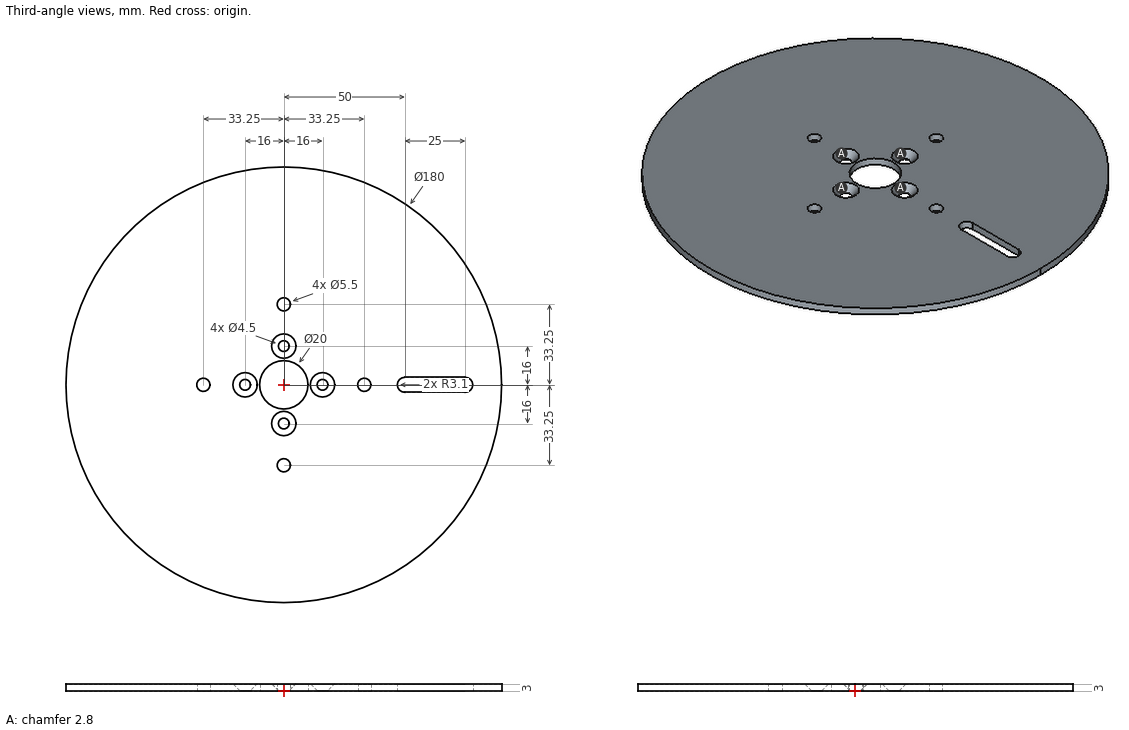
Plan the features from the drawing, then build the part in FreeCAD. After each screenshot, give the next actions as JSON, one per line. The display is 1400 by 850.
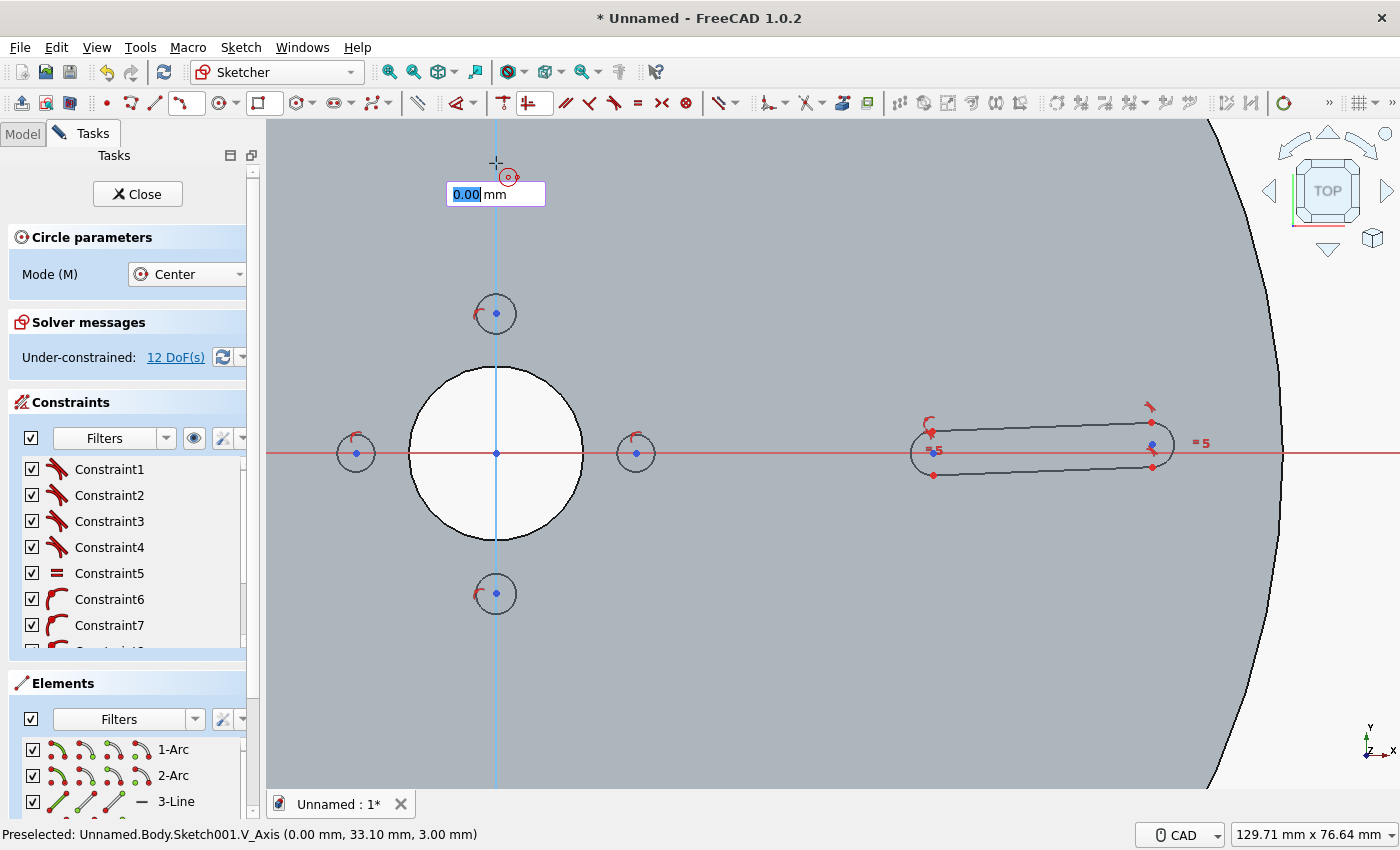
{"action": "scroll", "coordinate": [936, 455], "scroll_direction": "down", "scroll_amount": 2}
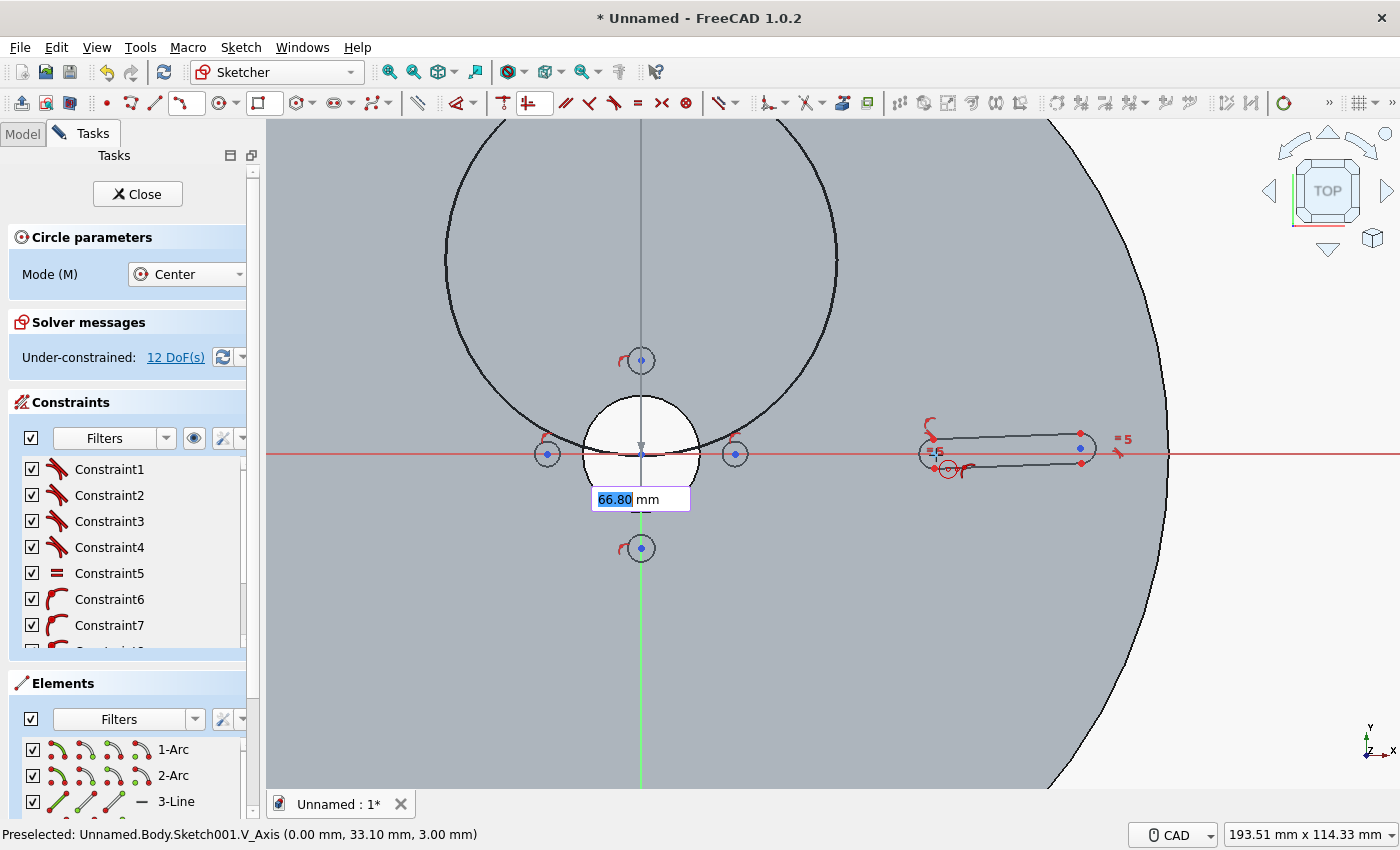
{"action": "scroll", "coordinate": [653, 248], "scroll_direction": "up", "scroll_amount": 2}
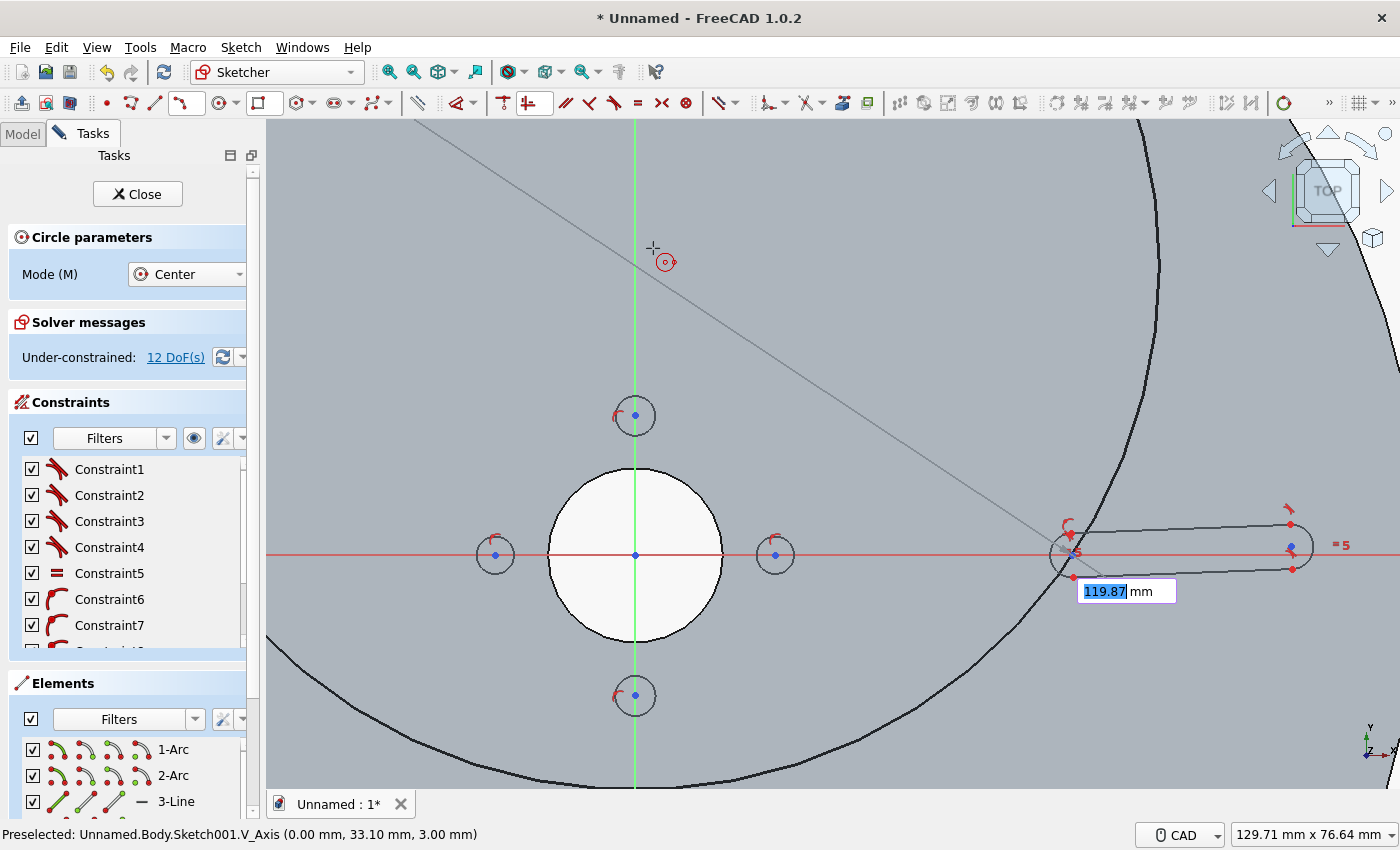
{"action": "left_click", "coordinate": [652, 248]}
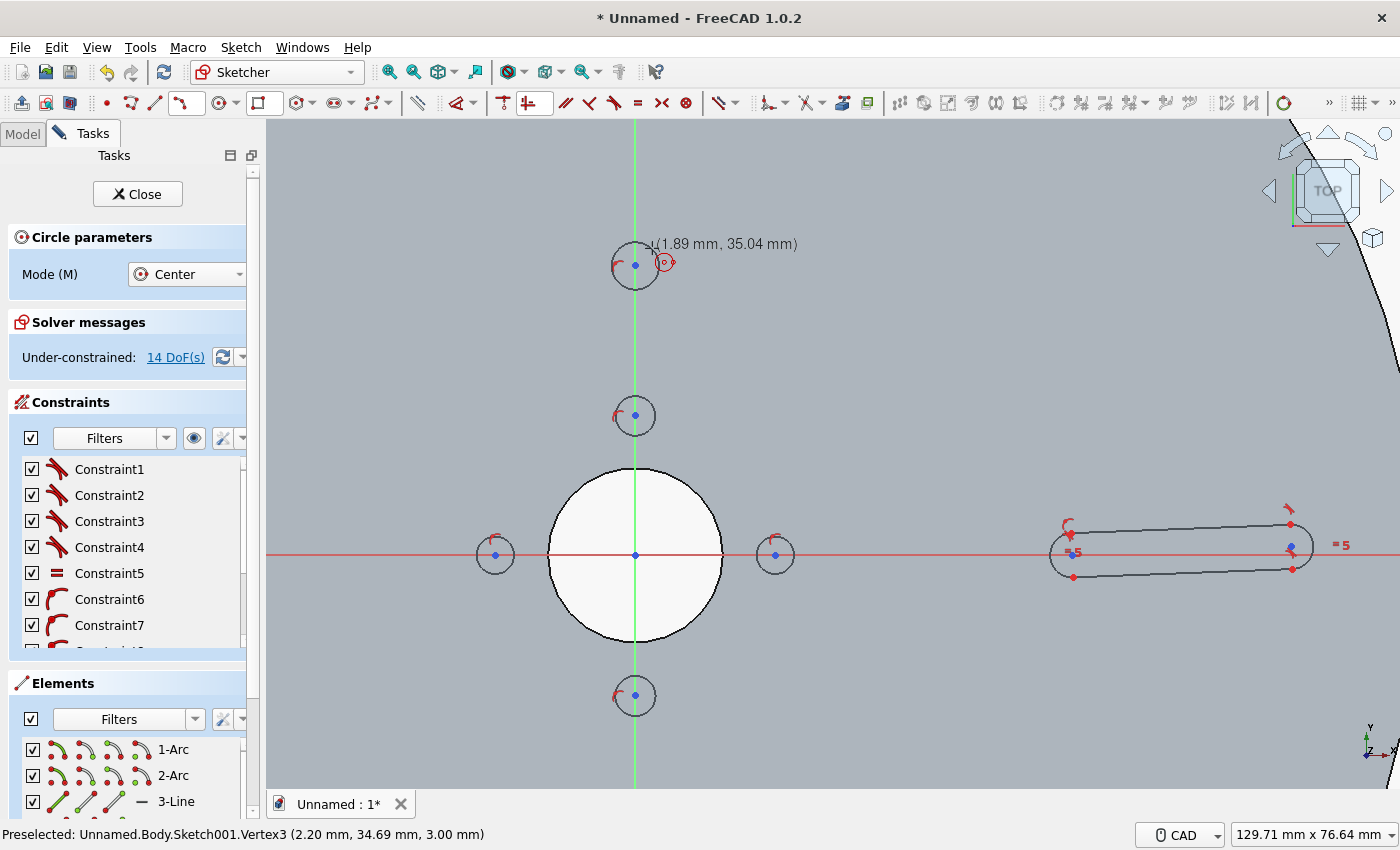
{"action": "left_click", "coordinate": [345, 555]}
{"action": "left_click", "coordinate": [362, 538]}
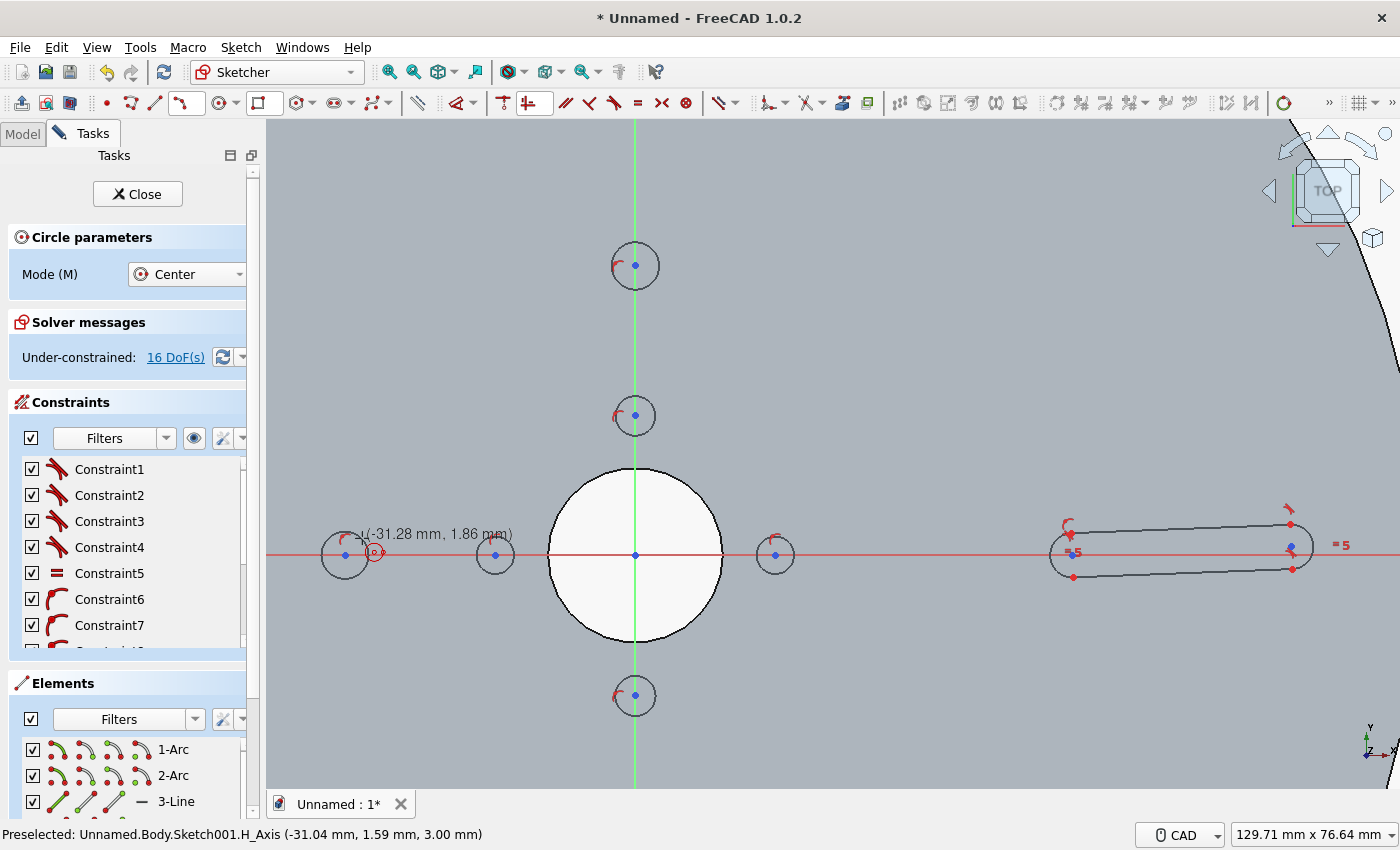
{"action": "scroll", "coordinate": [653, 248], "scroll_direction": "down", "scroll_amount": 2}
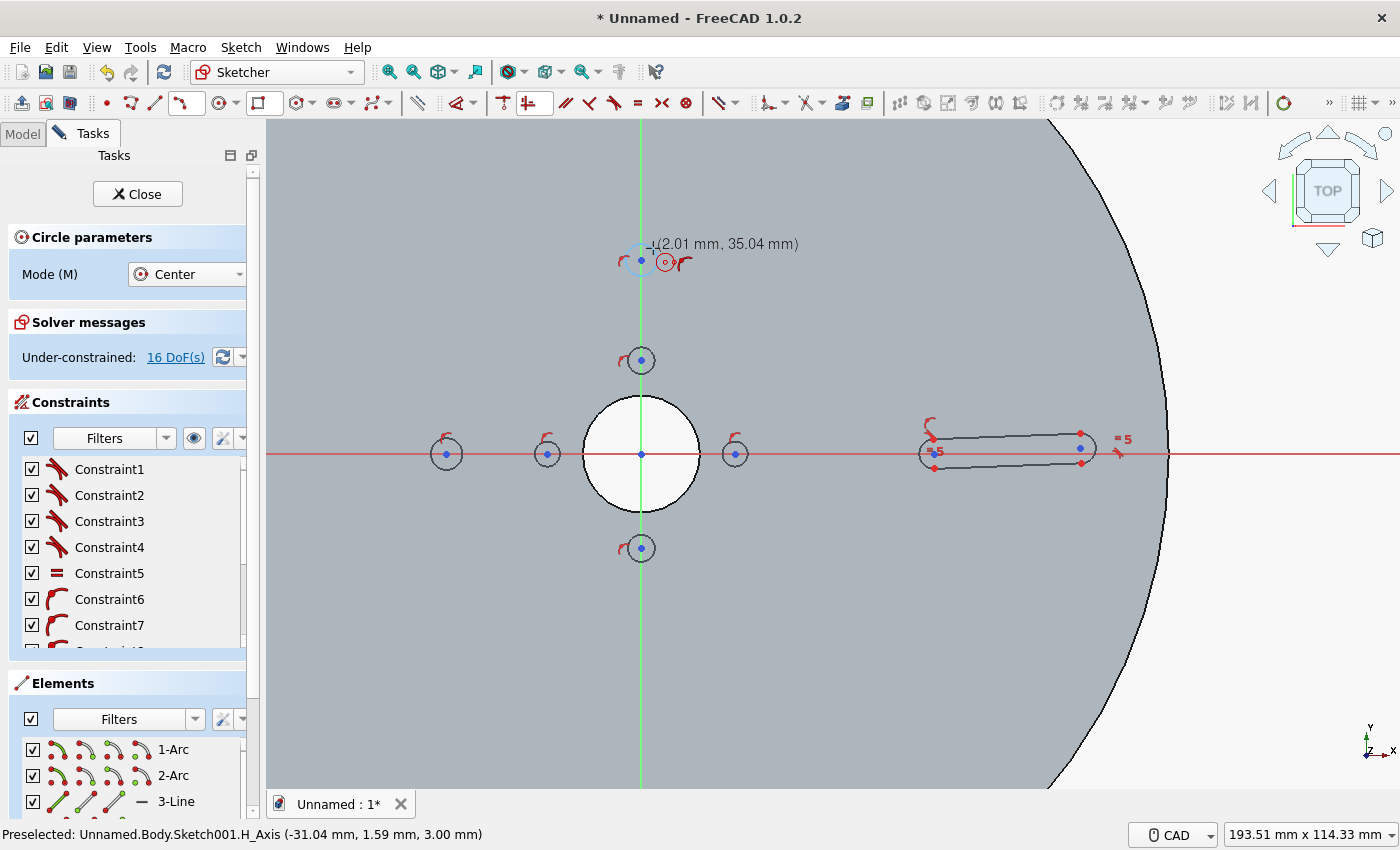
{"action": "scroll", "coordinate": [641, 649], "scroll_direction": "up", "scroll_amount": 2}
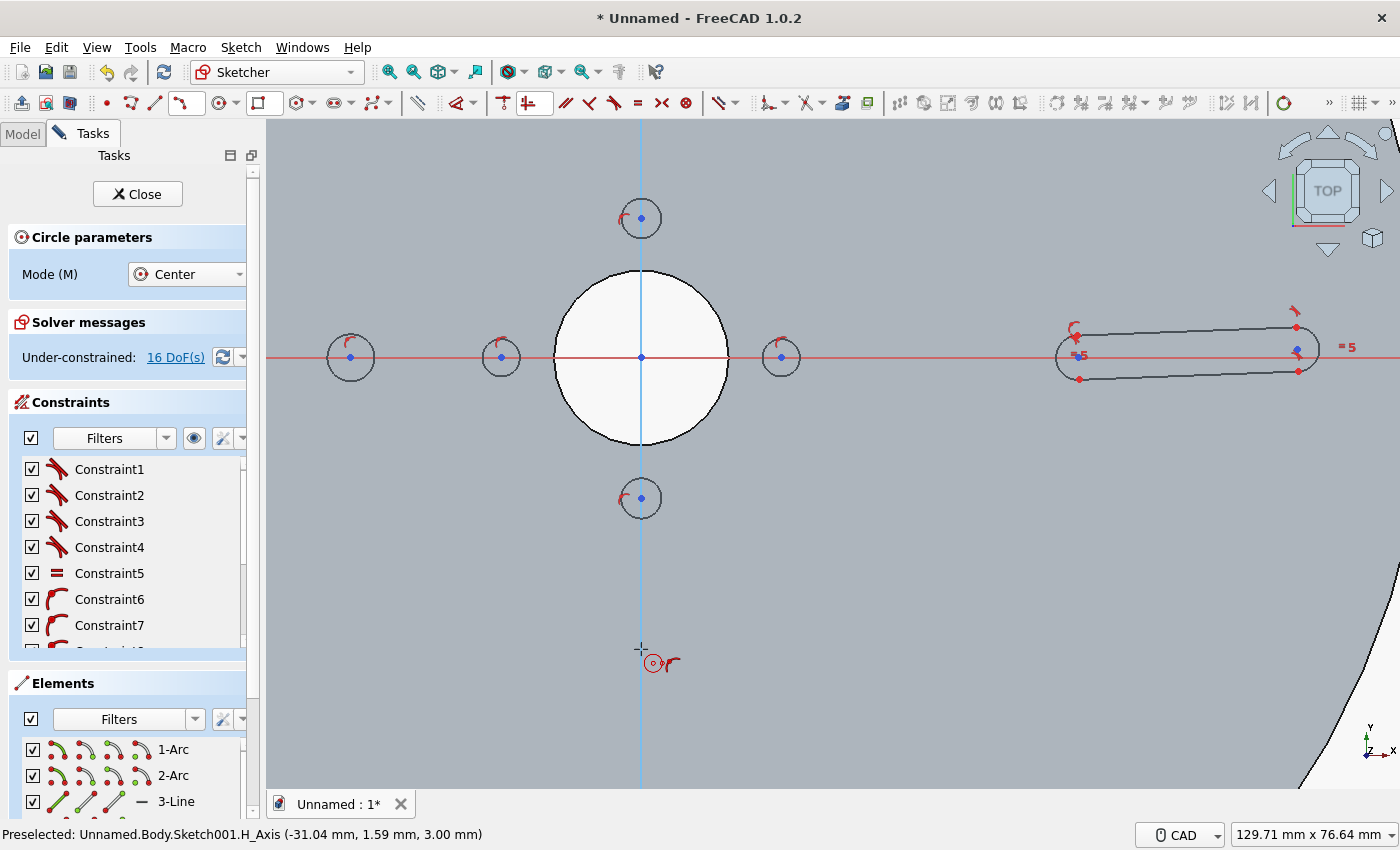
{"action": "left_click", "coordinate": [641, 648]}
{"action": "left_click", "coordinate": [658, 631]}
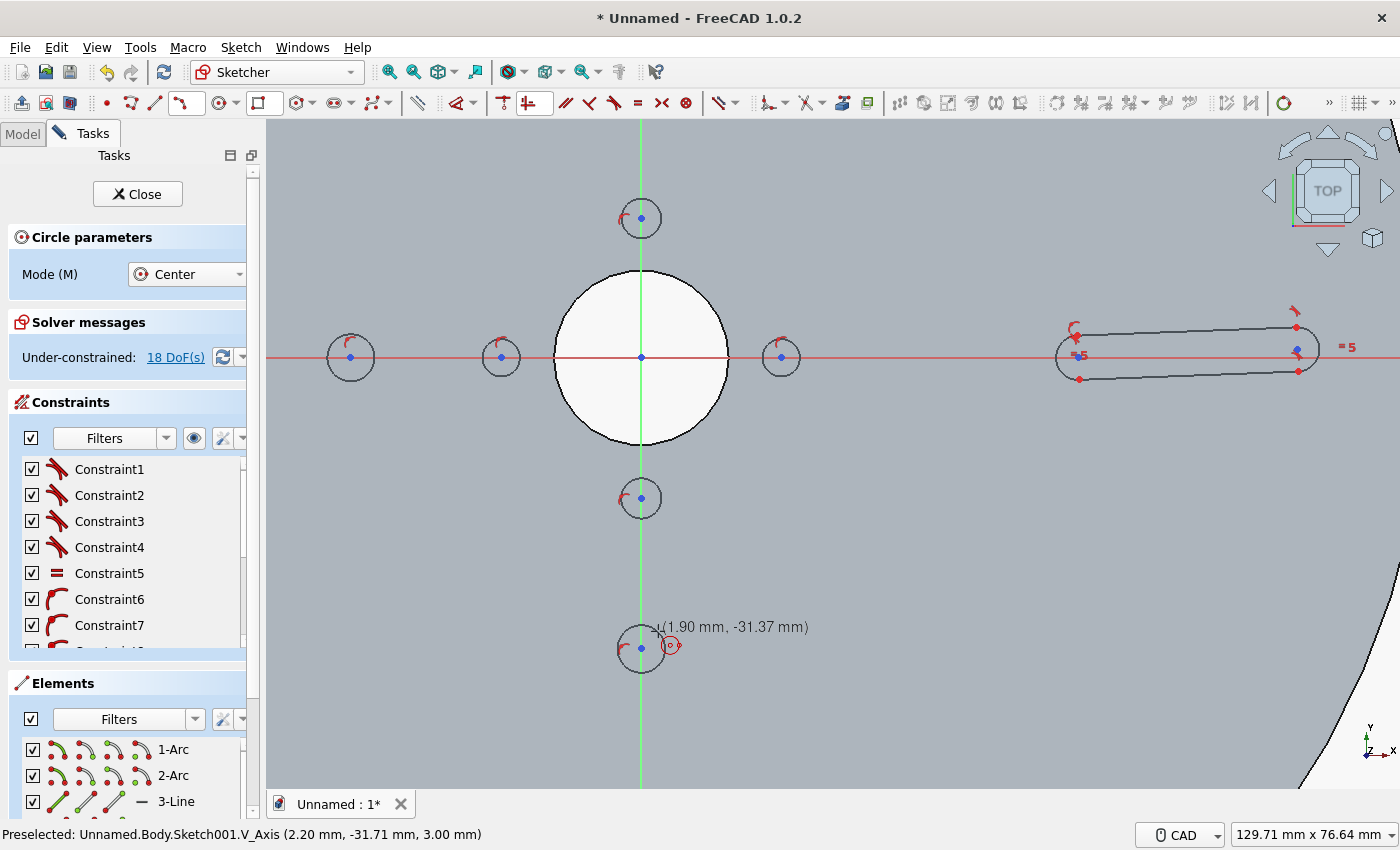
{"action": "left_click", "coordinate": [932, 358]}
{"action": "left_click", "coordinate": [949, 341]}
{"action": "key", "text": "Escape"}